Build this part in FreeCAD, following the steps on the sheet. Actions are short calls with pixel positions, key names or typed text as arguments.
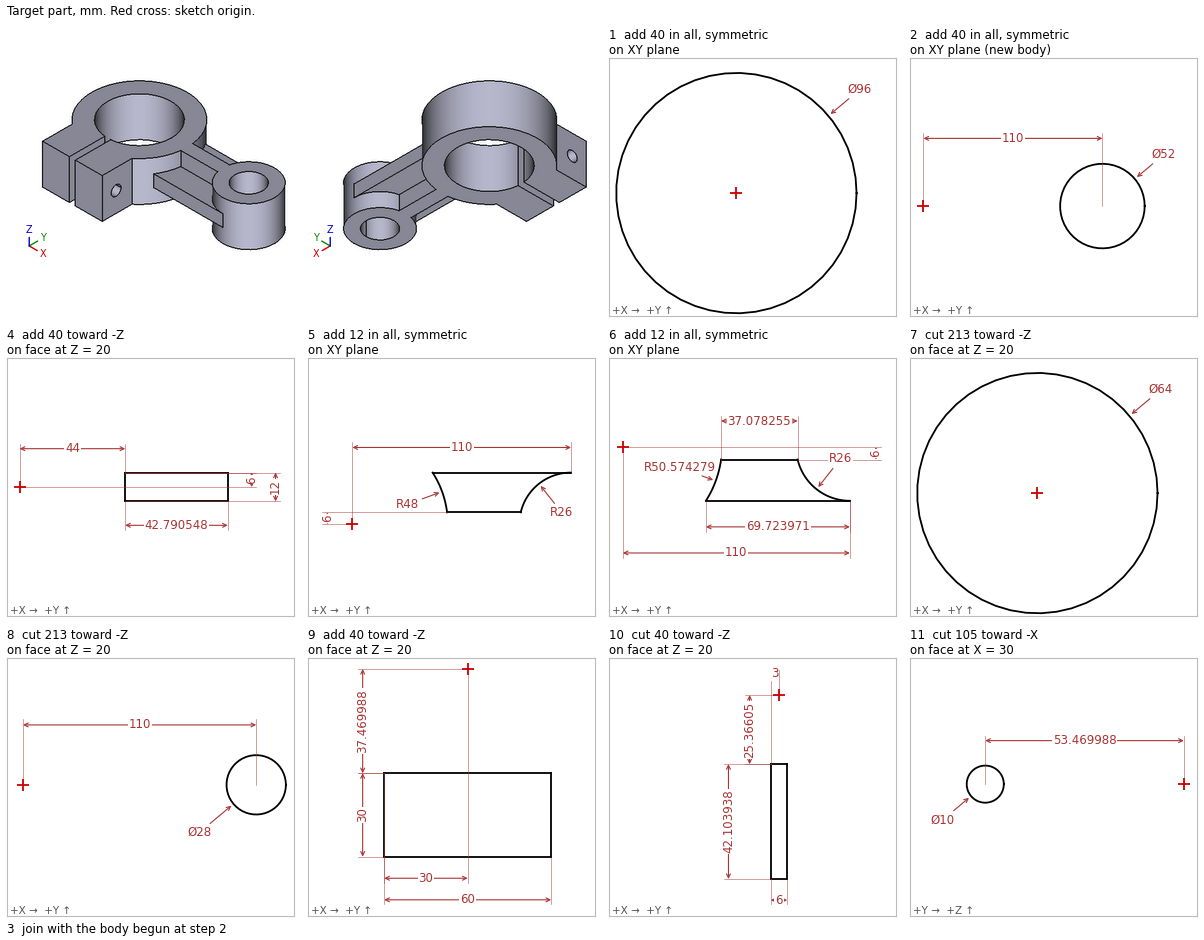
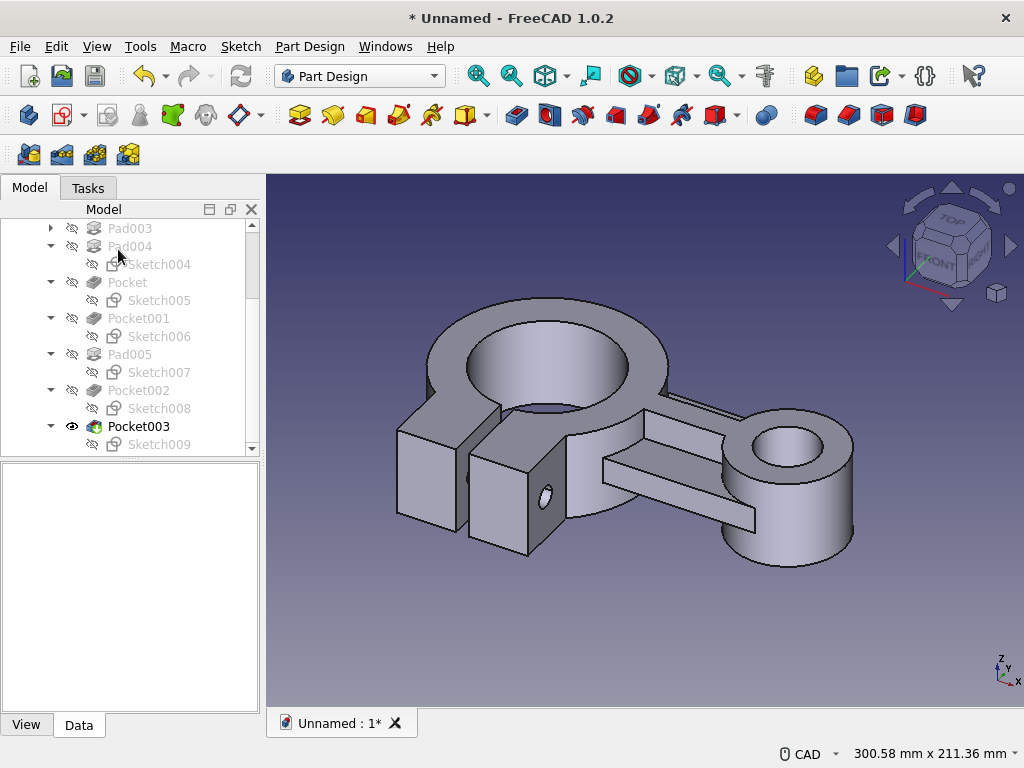
key(0)